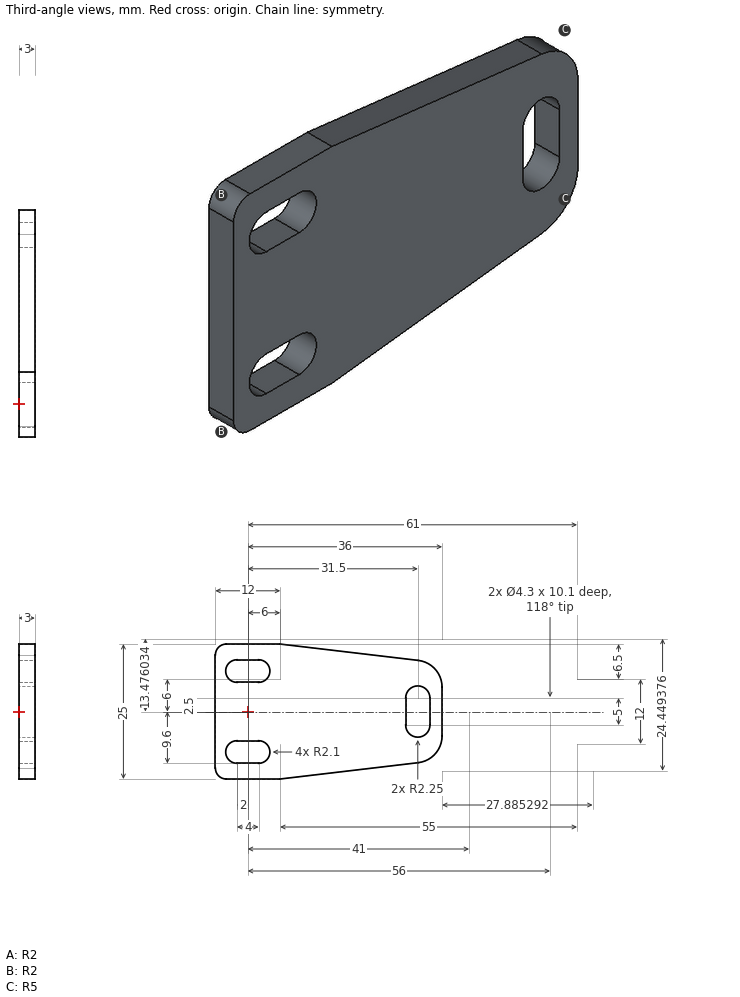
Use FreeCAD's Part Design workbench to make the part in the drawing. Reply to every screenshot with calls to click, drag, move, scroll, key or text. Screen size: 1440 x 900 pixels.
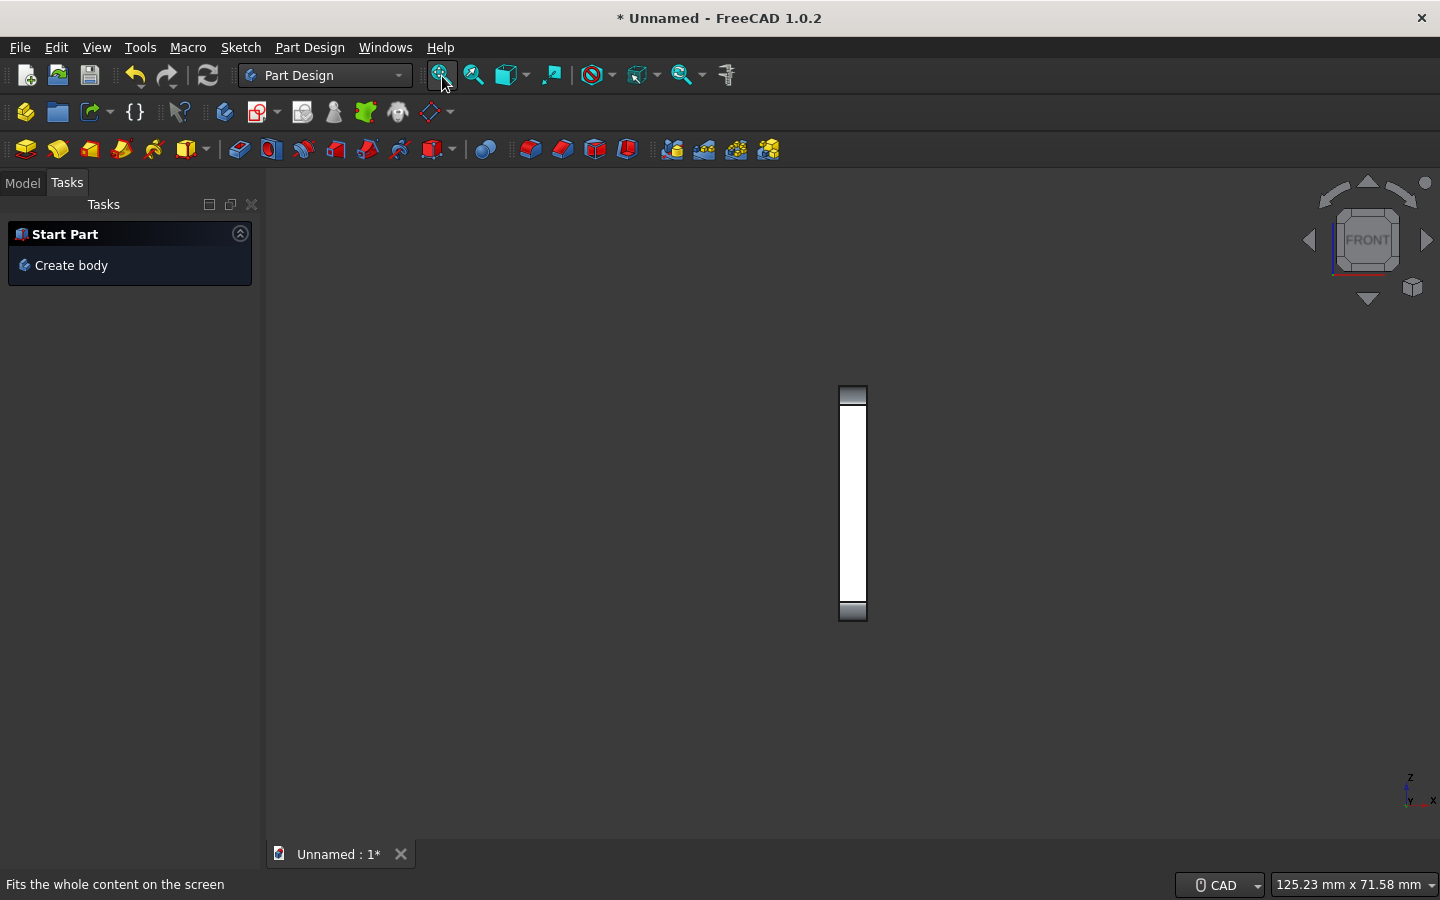
click(258, 112)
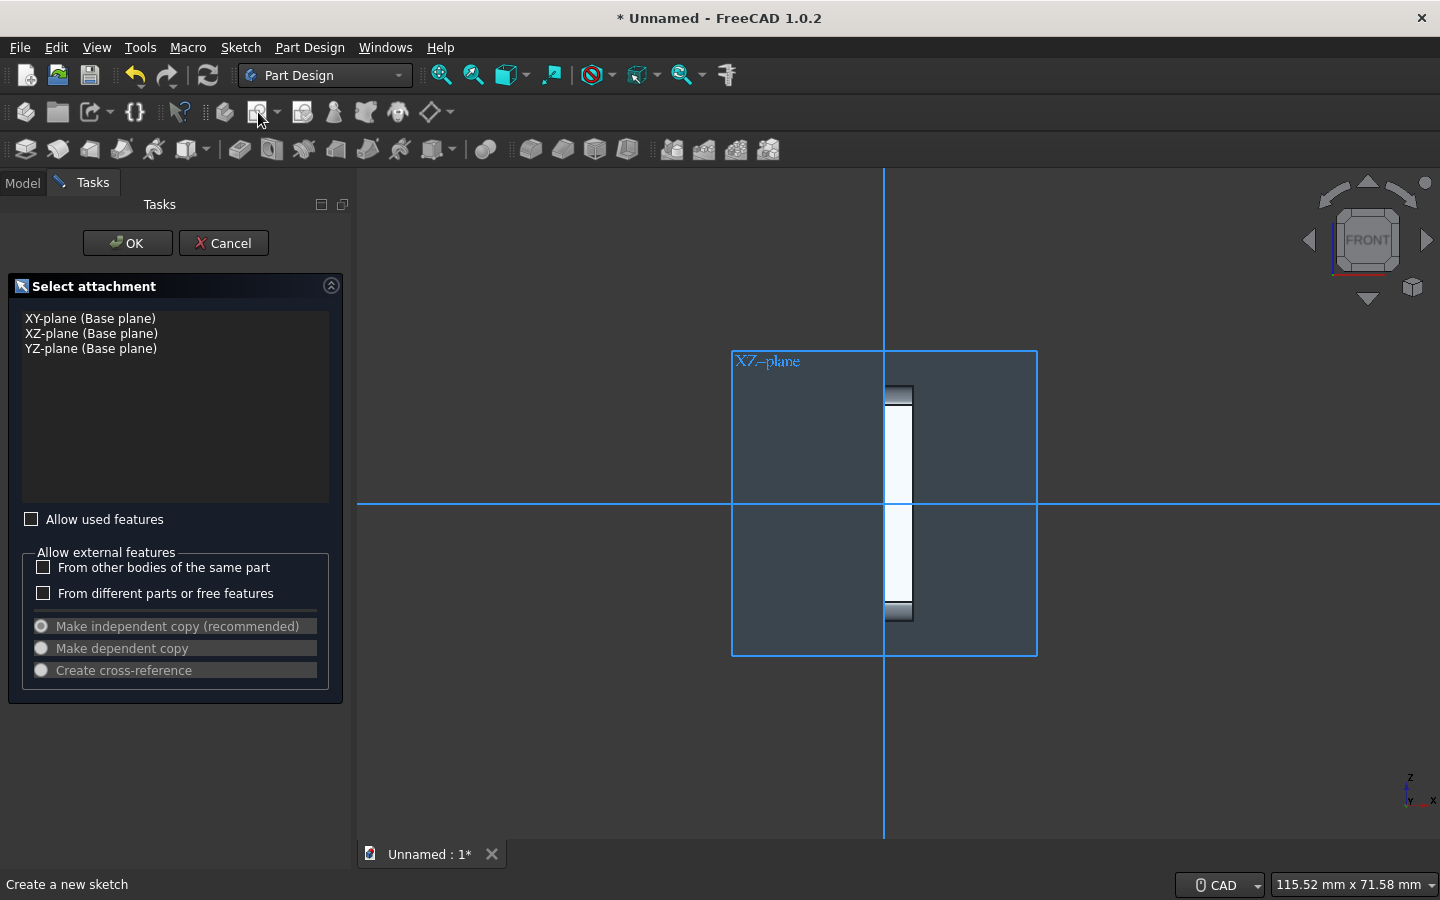
click(82, 348)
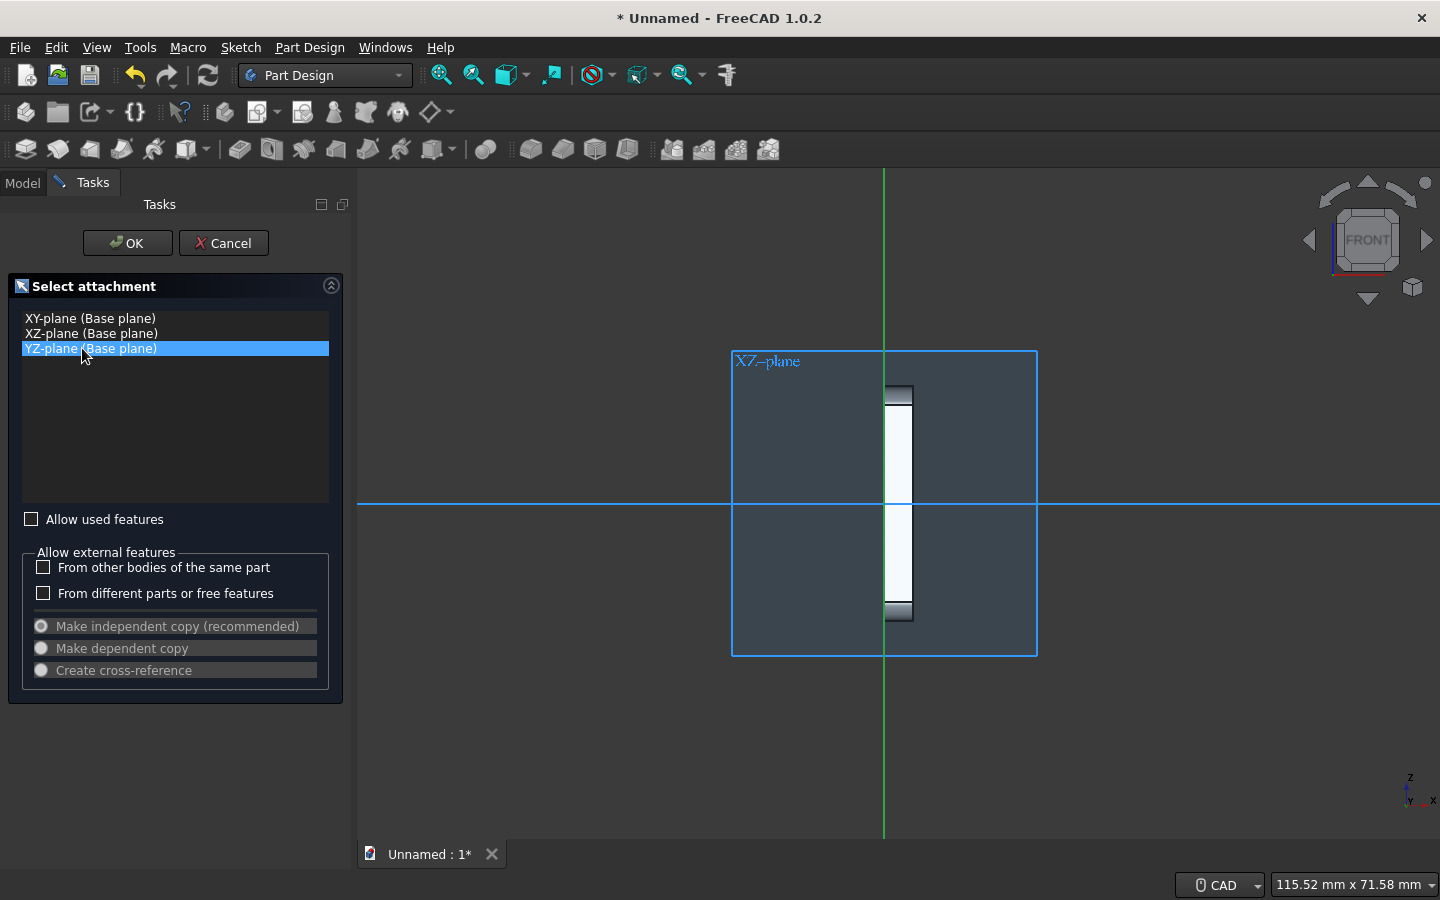
click(128, 243)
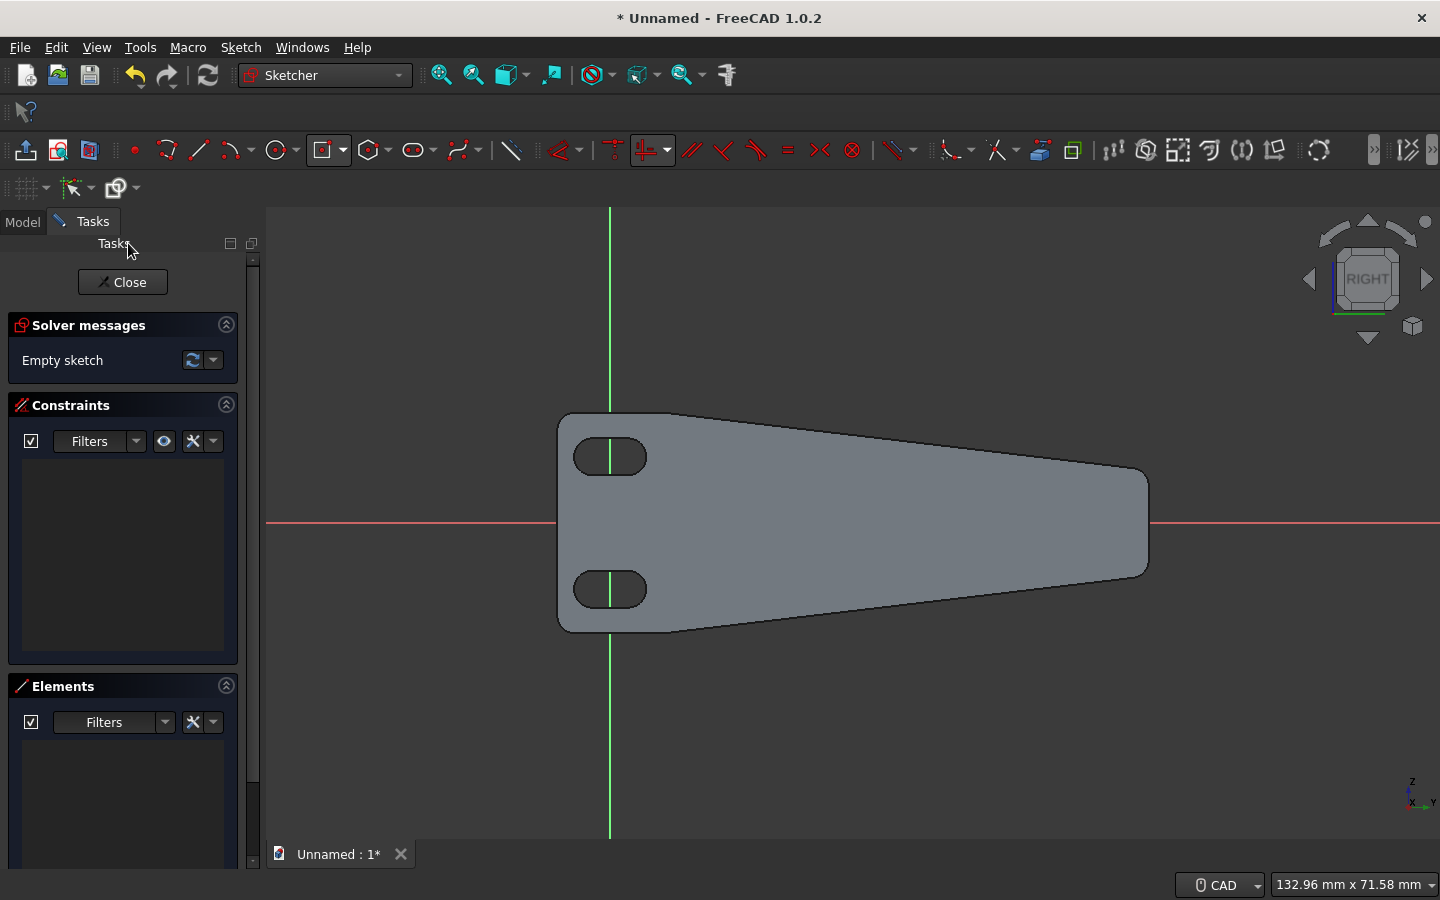
click(90, 150)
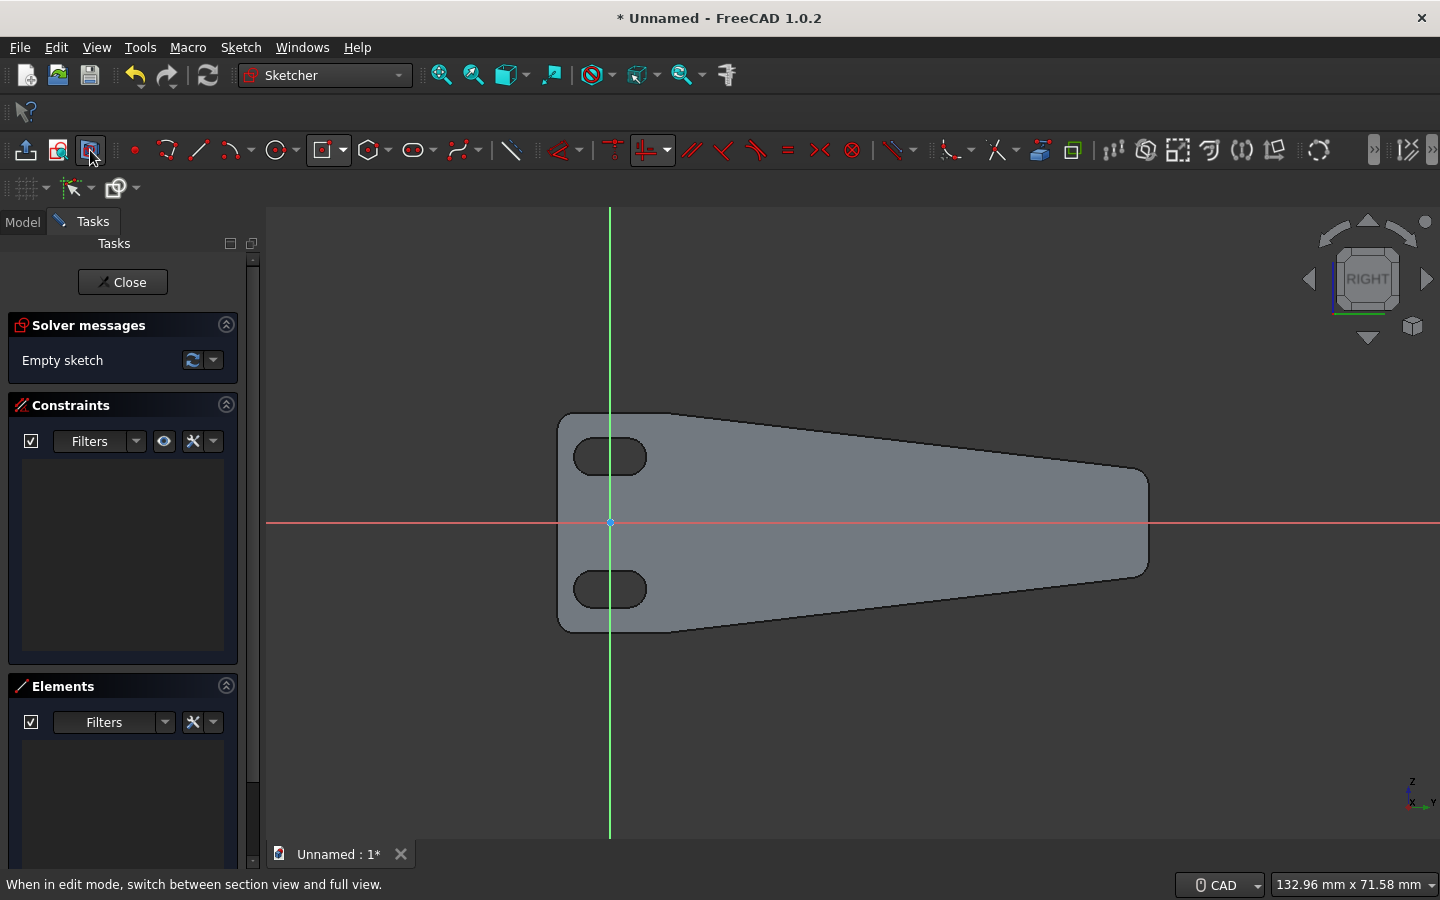
scroll(1122, 523, up, 7)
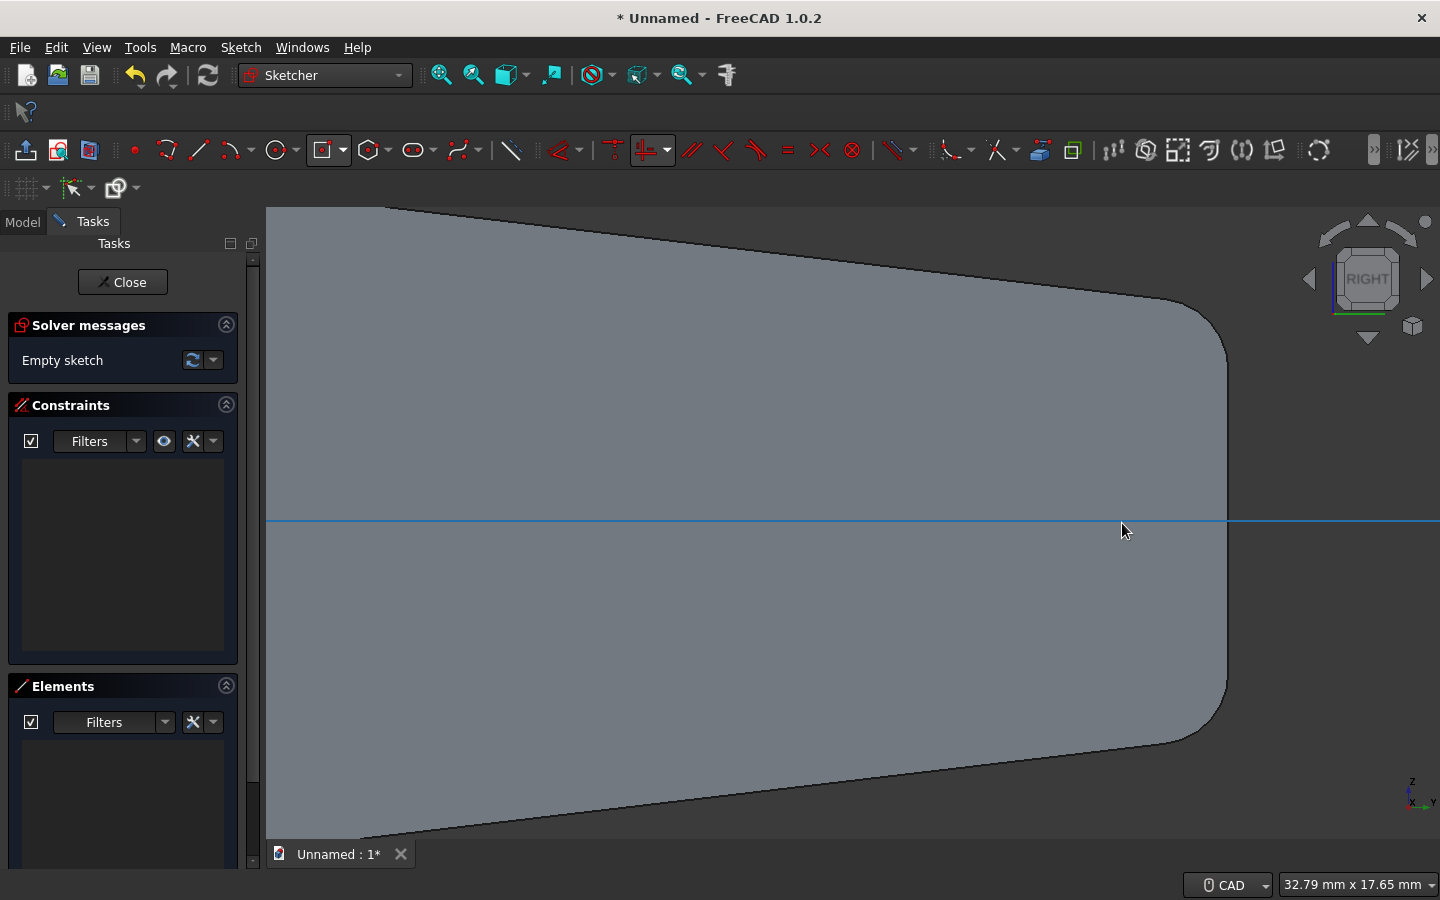
key(g)
key(c)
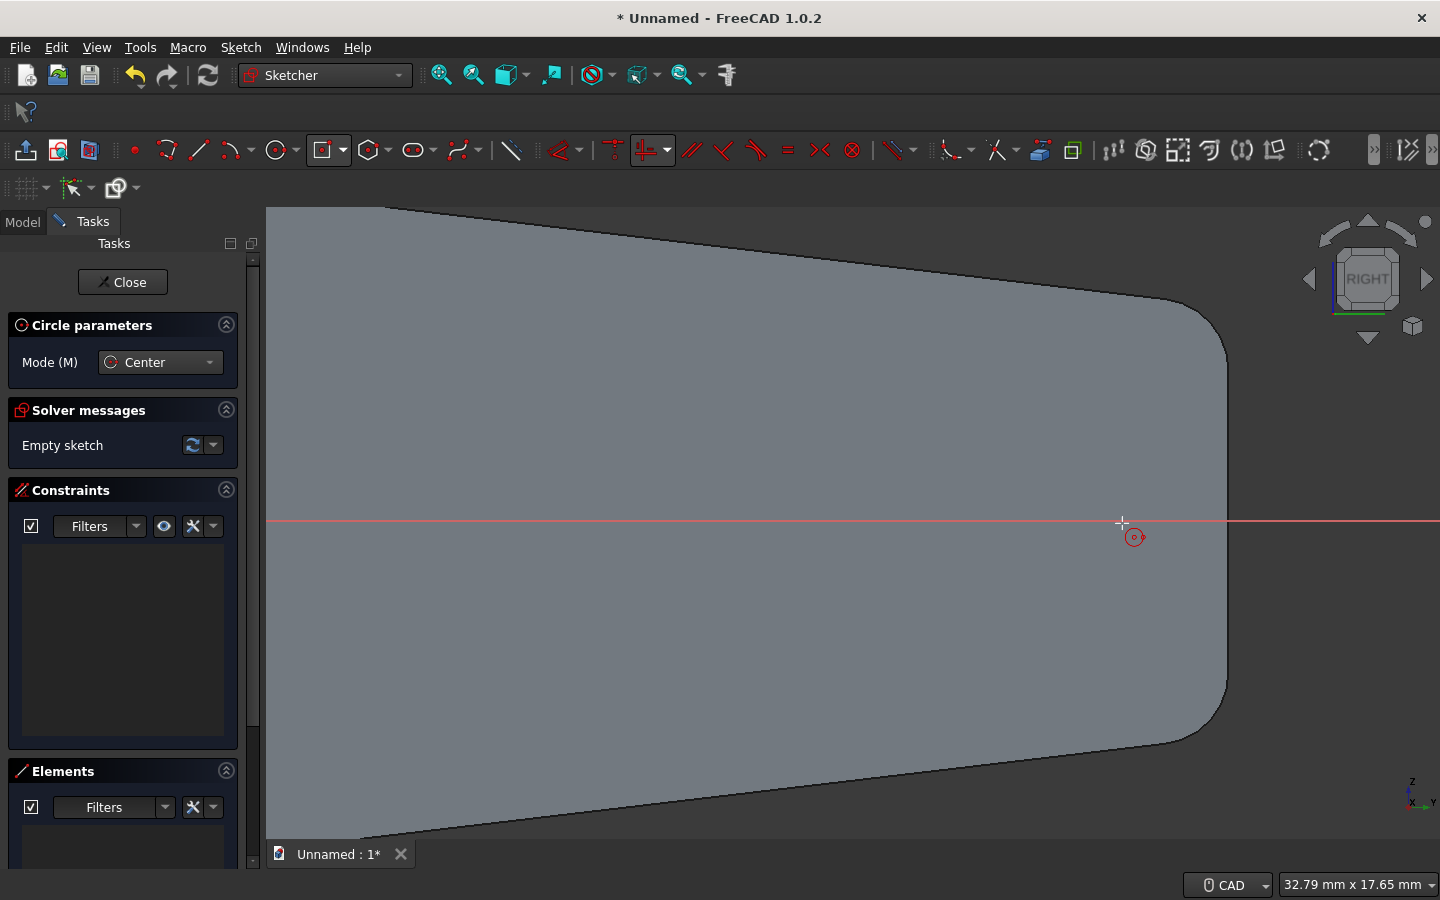
click(1049, 521)
click(1104, 467)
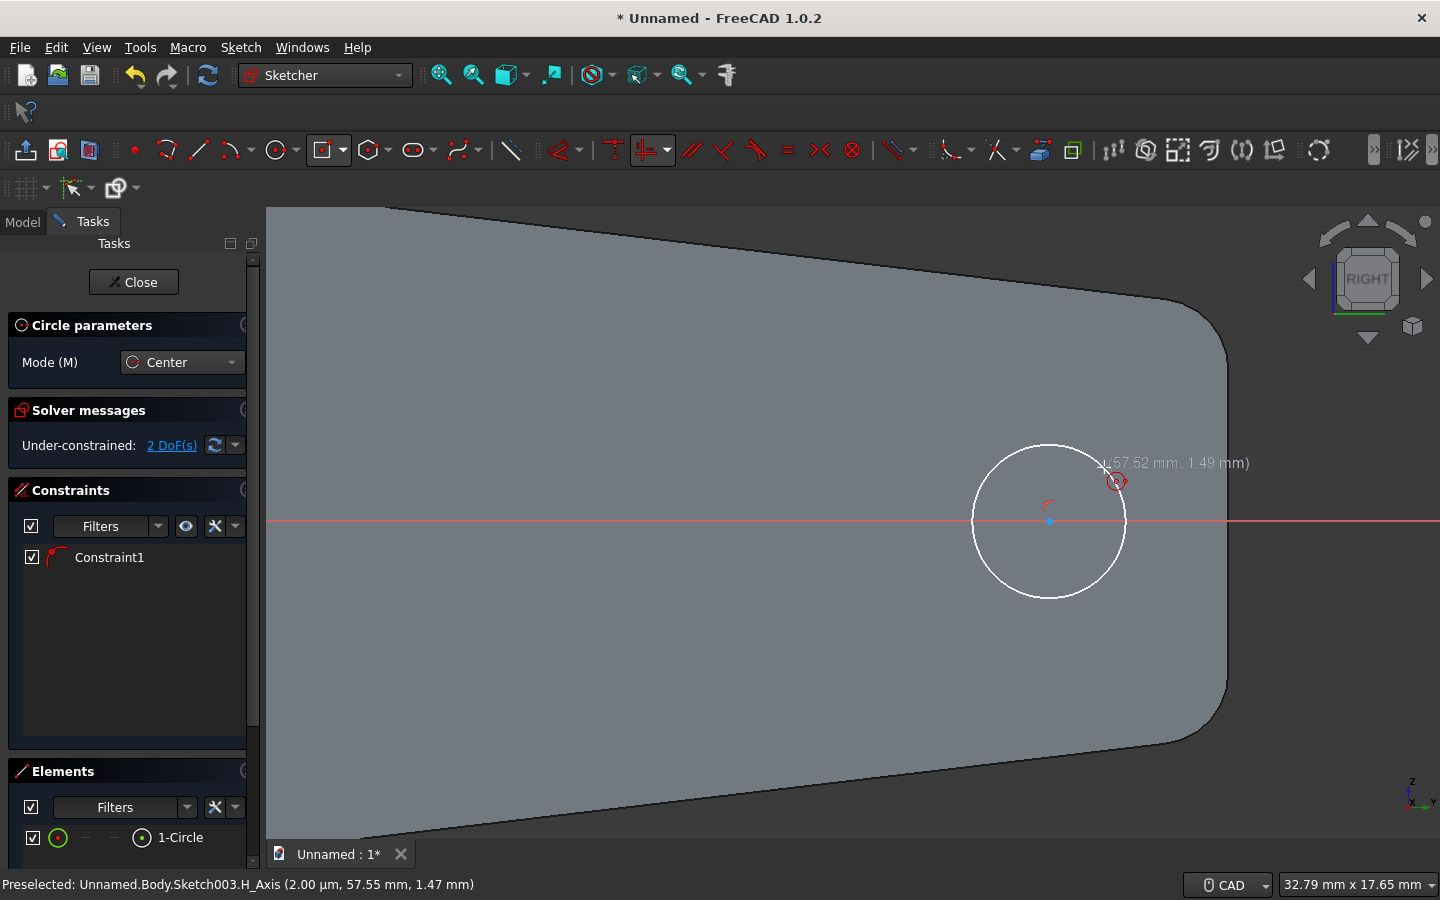
click(512, 521)
click(567, 467)
key(Escape)